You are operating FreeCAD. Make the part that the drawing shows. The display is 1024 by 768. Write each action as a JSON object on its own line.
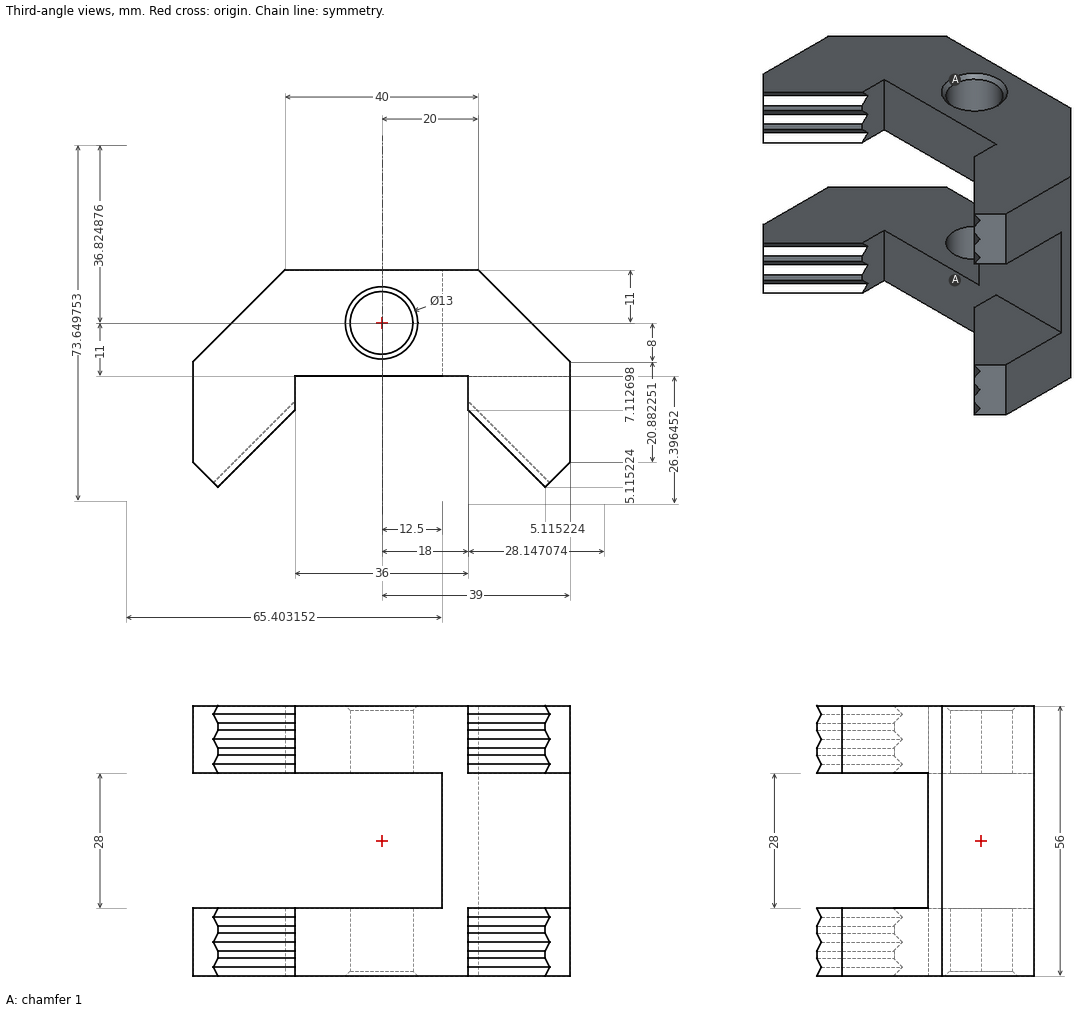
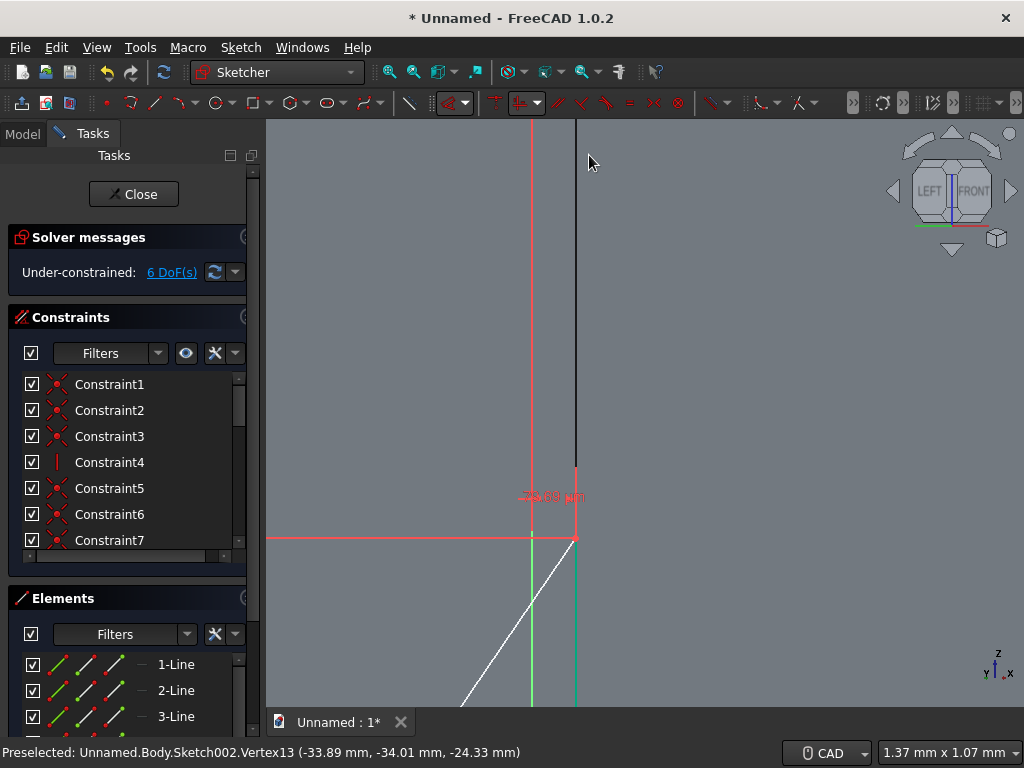
{"action": "scroll", "coordinate": [587, 570], "scroll_direction": "down", "scroll_amount": 18}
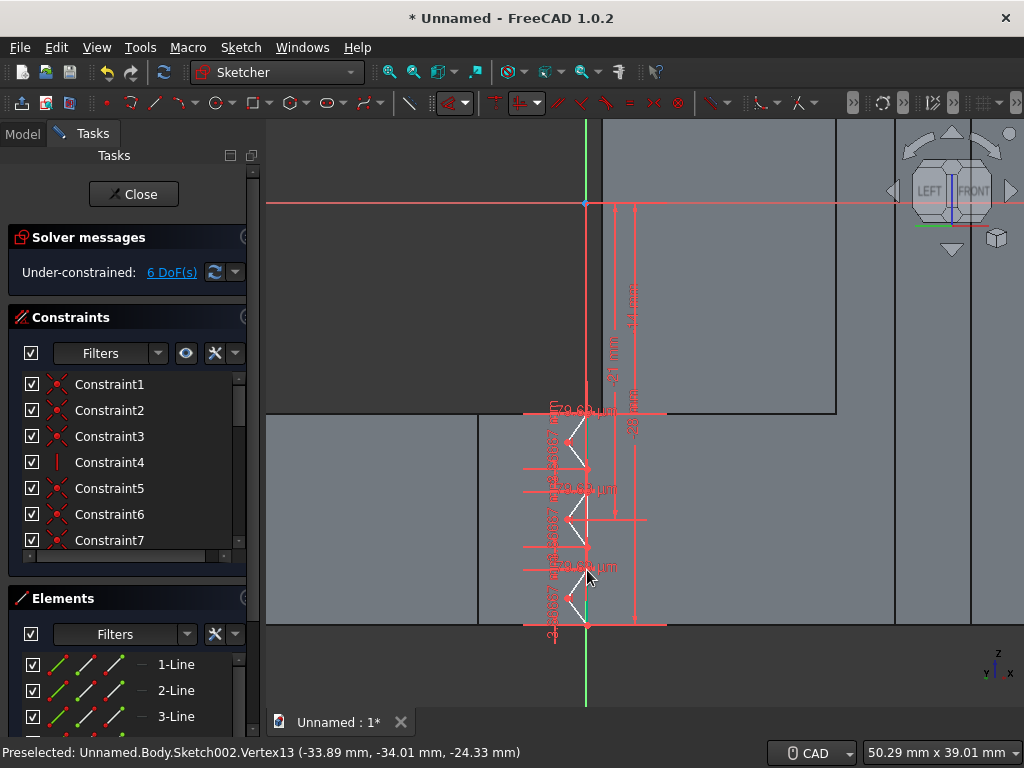
{"action": "scroll", "coordinate": [567, 520], "scroll_direction": "up", "scroll_amount": 4}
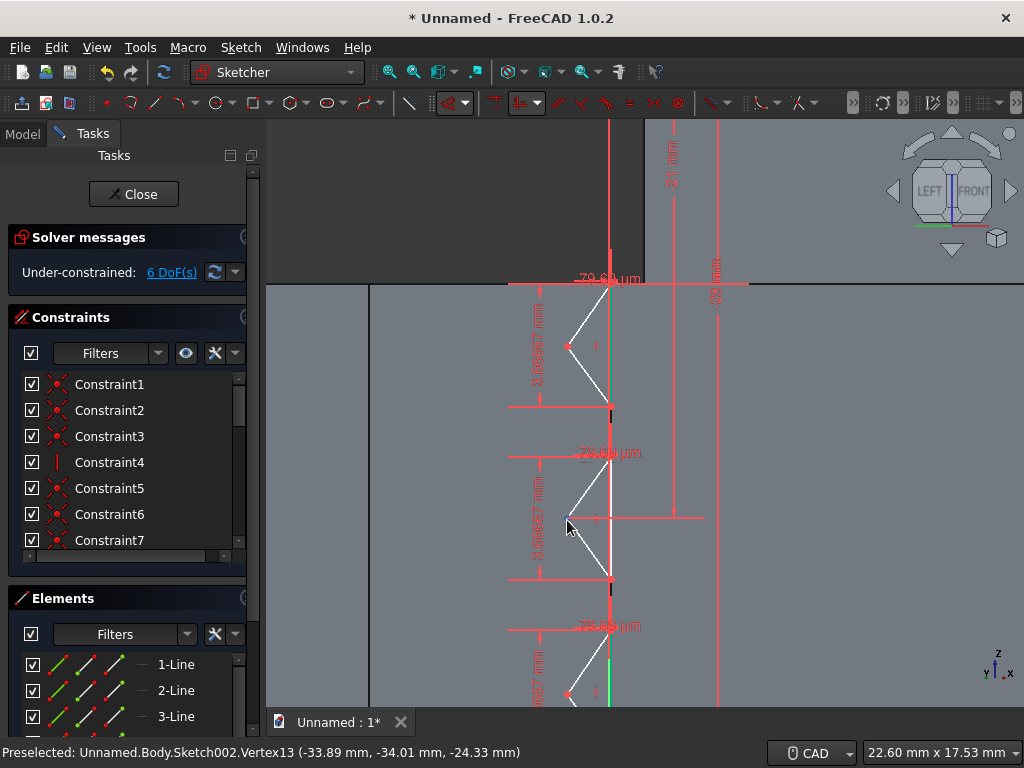
{"action": "left_click", "coordinate": [567, 518]}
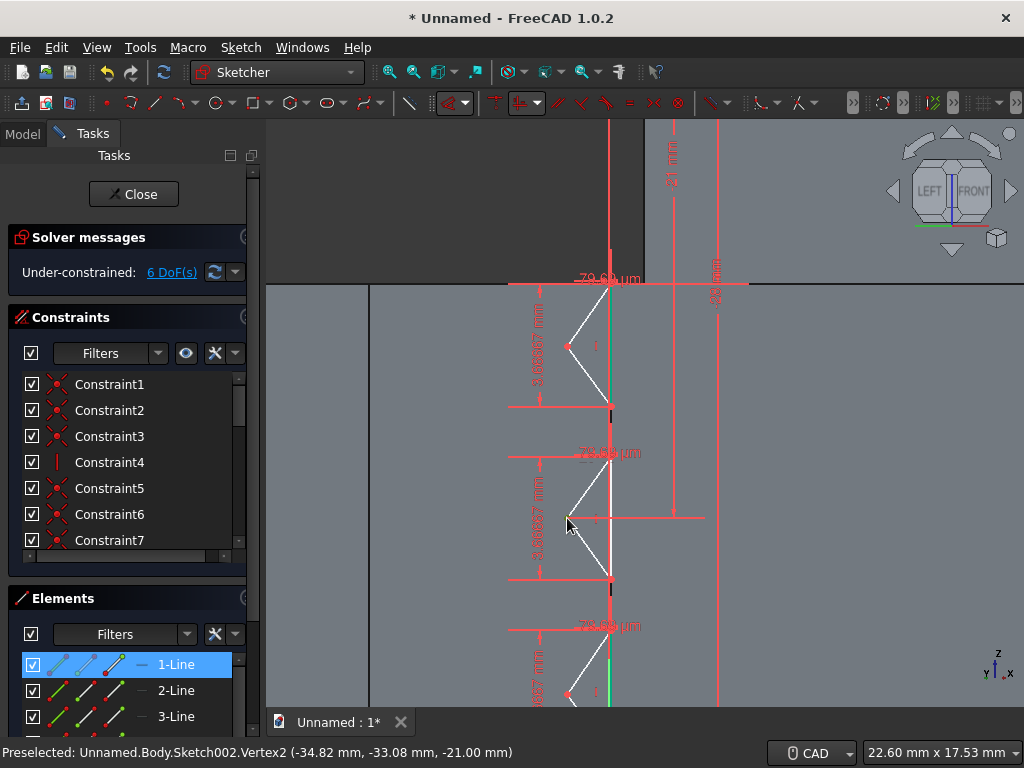
{"action": "key", "text": "l"}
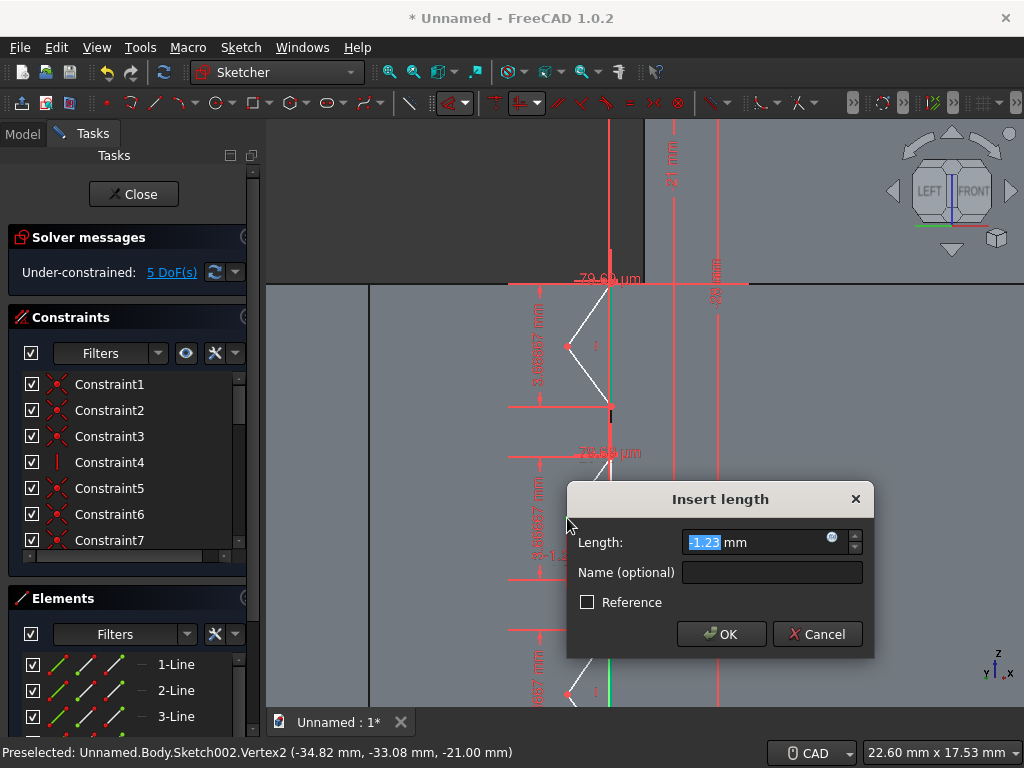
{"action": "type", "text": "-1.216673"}
{"action": "key", "text": "Return"}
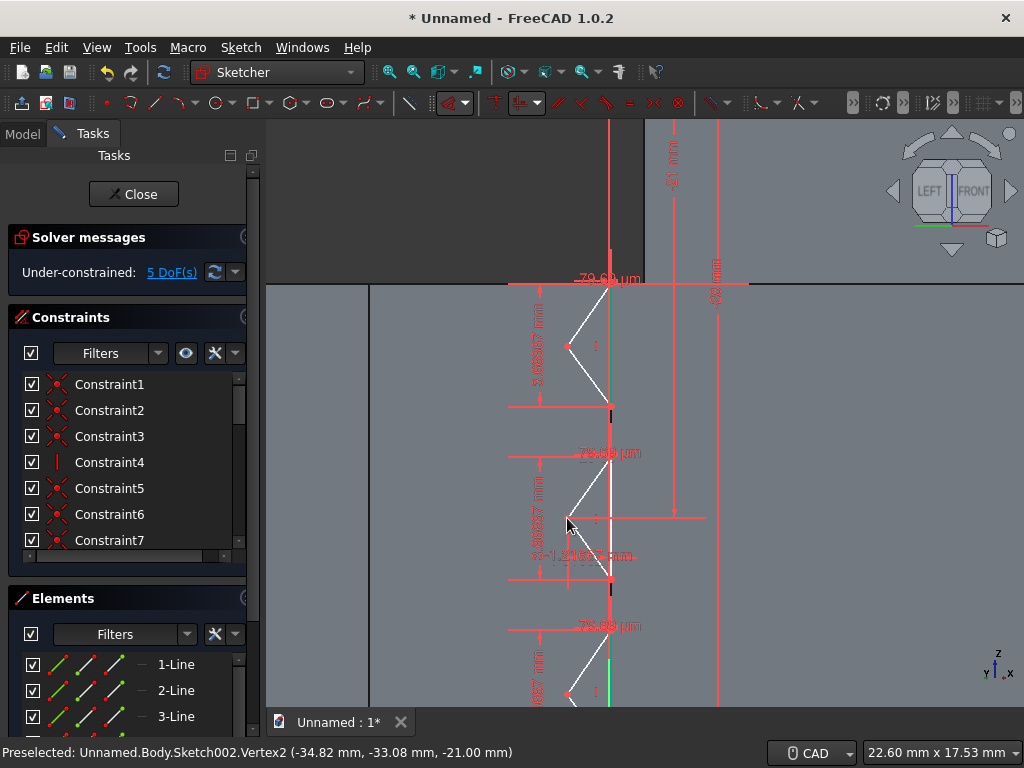
{"action": "left_click", "coordinate": [567, 347]}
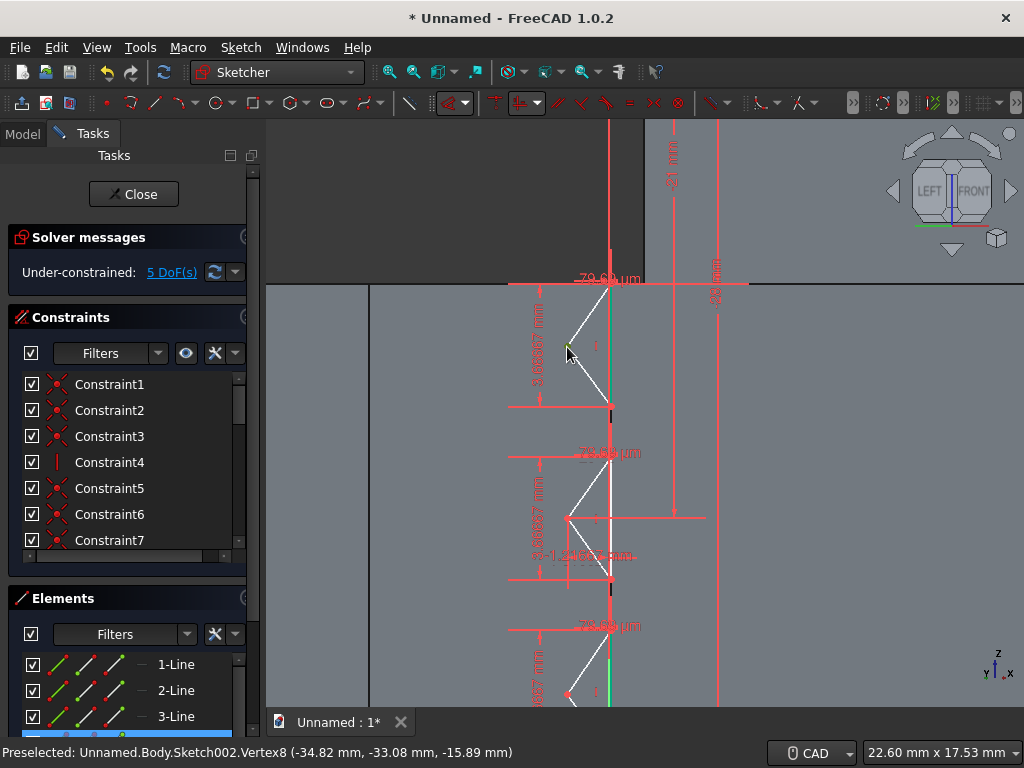
{"action": "left_click", "coordinate": [468, 104]}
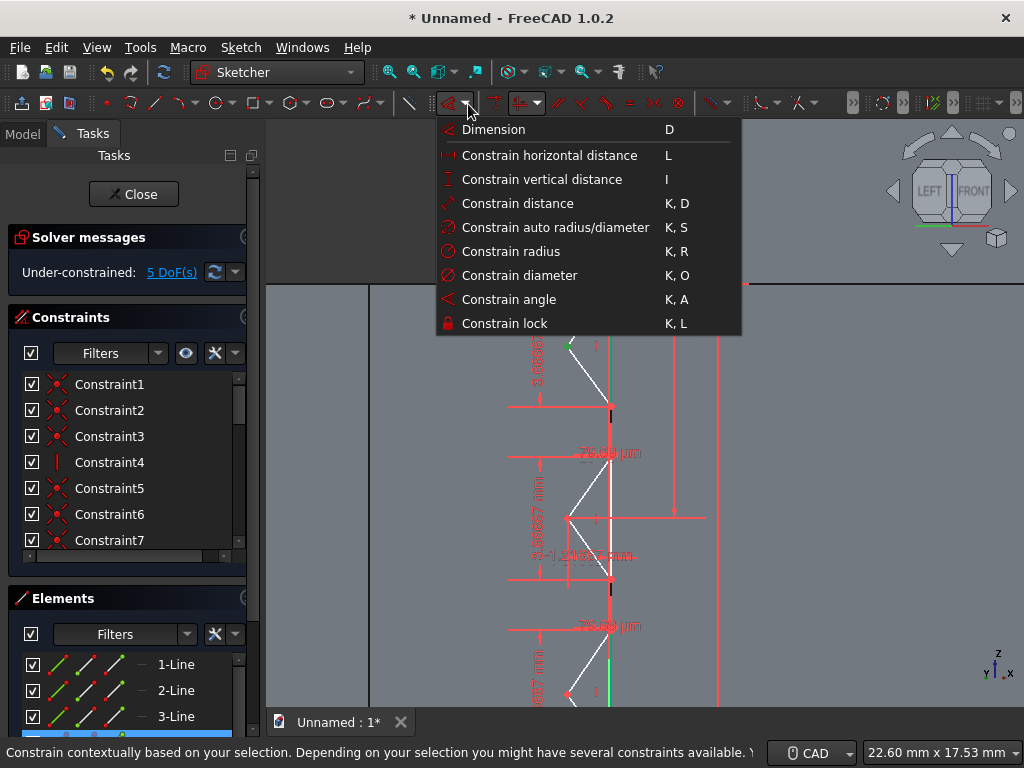
{"action": "left_click", "coordinate": [589, 155]}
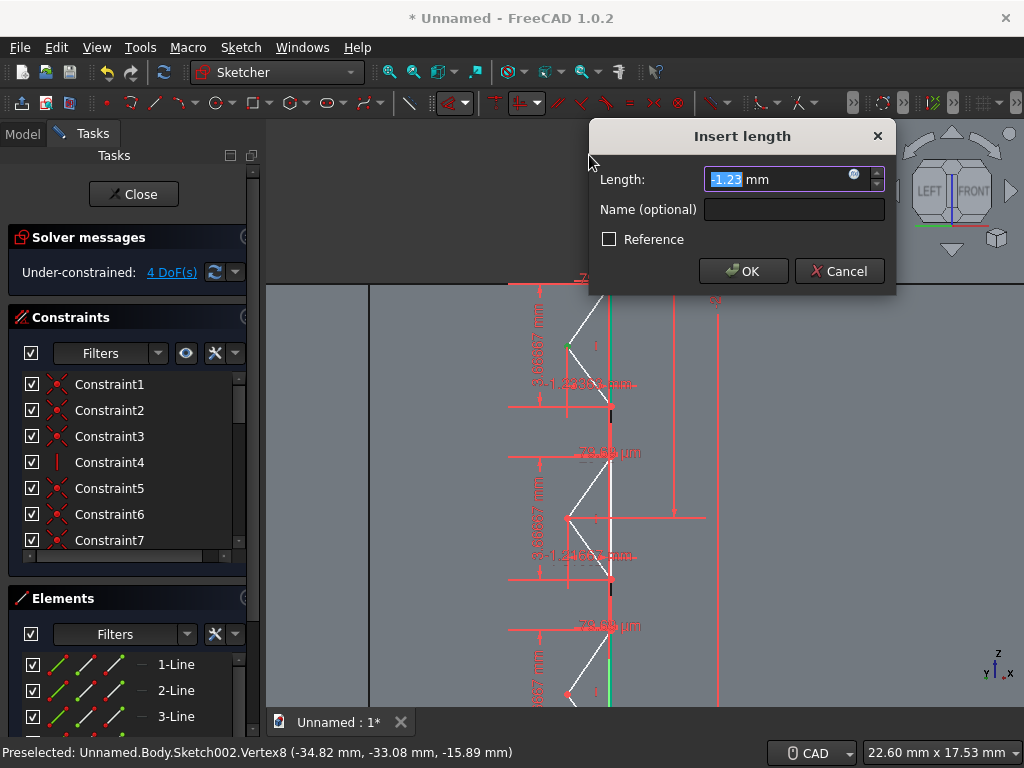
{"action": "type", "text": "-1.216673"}
{"action": "key", "text": "Return"}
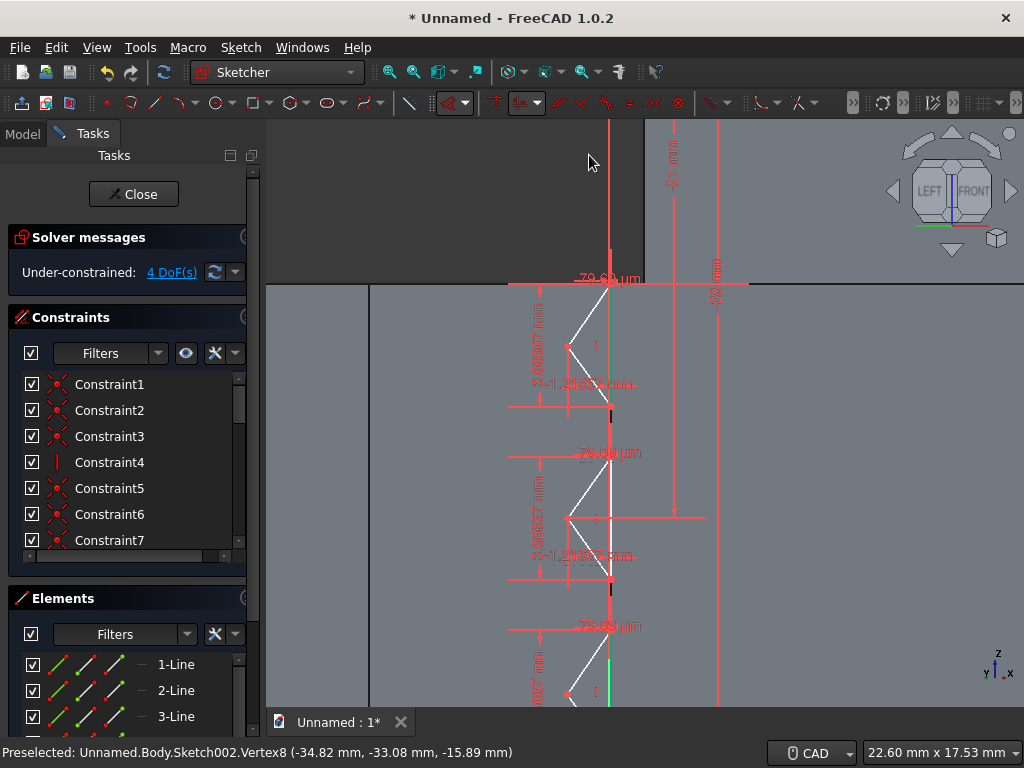
{"action": "scroll", "coordinate": [569, 488], "scroll_direction": "down", "scroll_amount": 5}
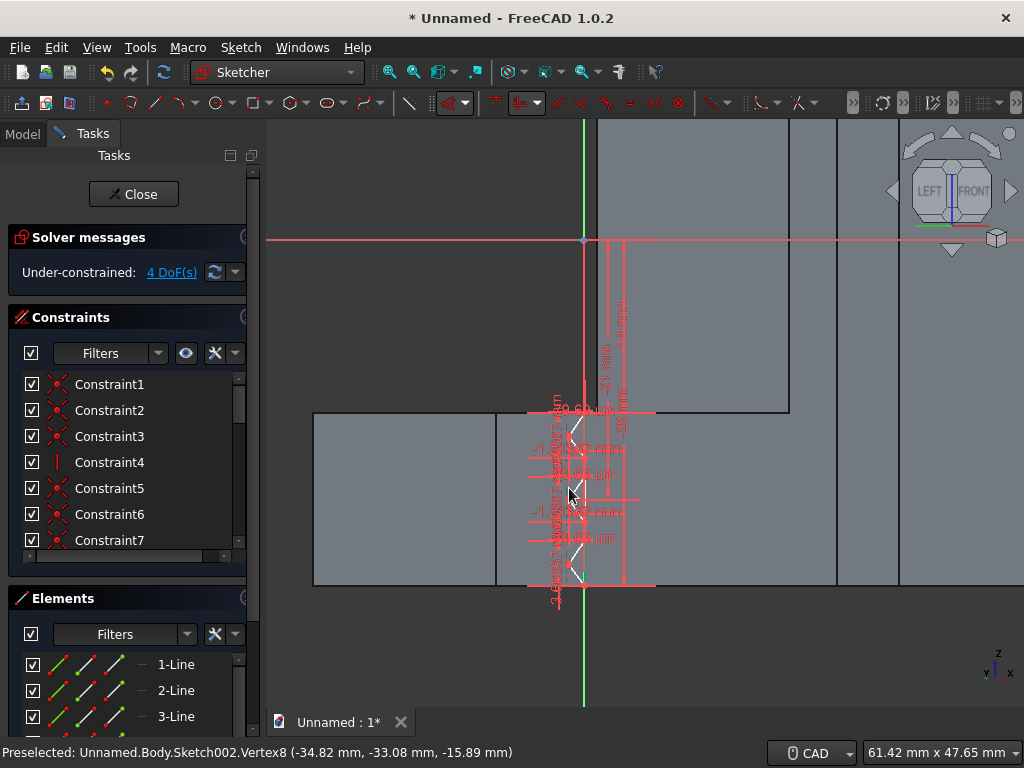
{"action": "scroll", "coordinate": [569, 564], "scroll_direction": "up", "scroll_amount": 5}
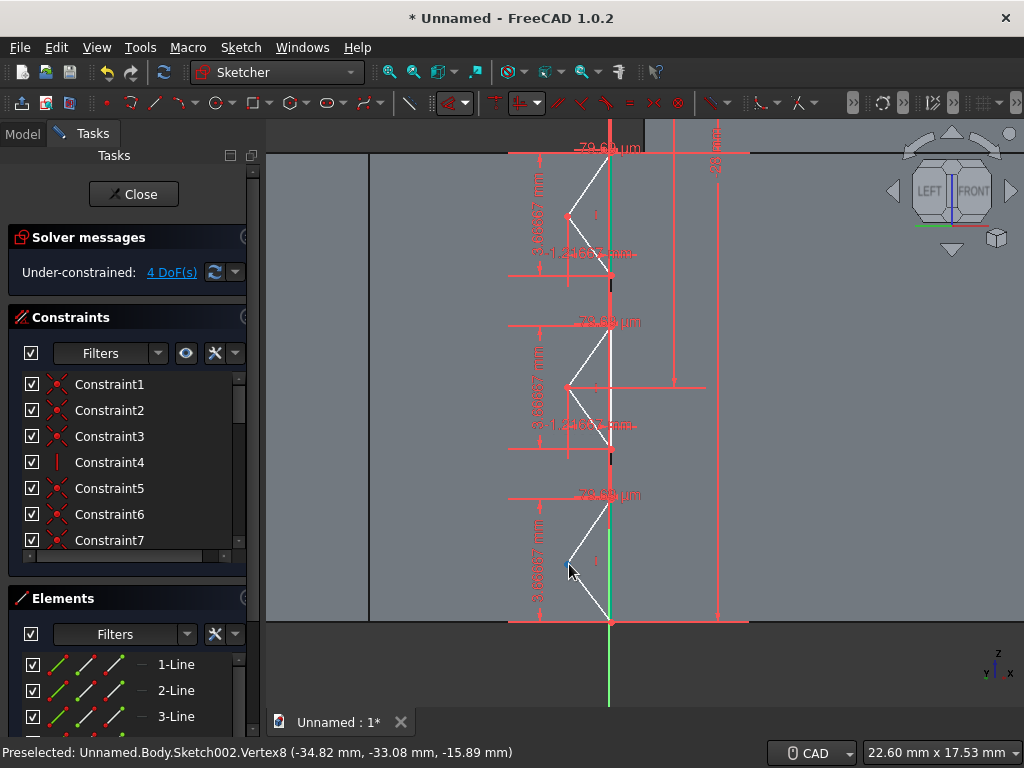
{"action": "left_click", "coordinate": [567, 564]}